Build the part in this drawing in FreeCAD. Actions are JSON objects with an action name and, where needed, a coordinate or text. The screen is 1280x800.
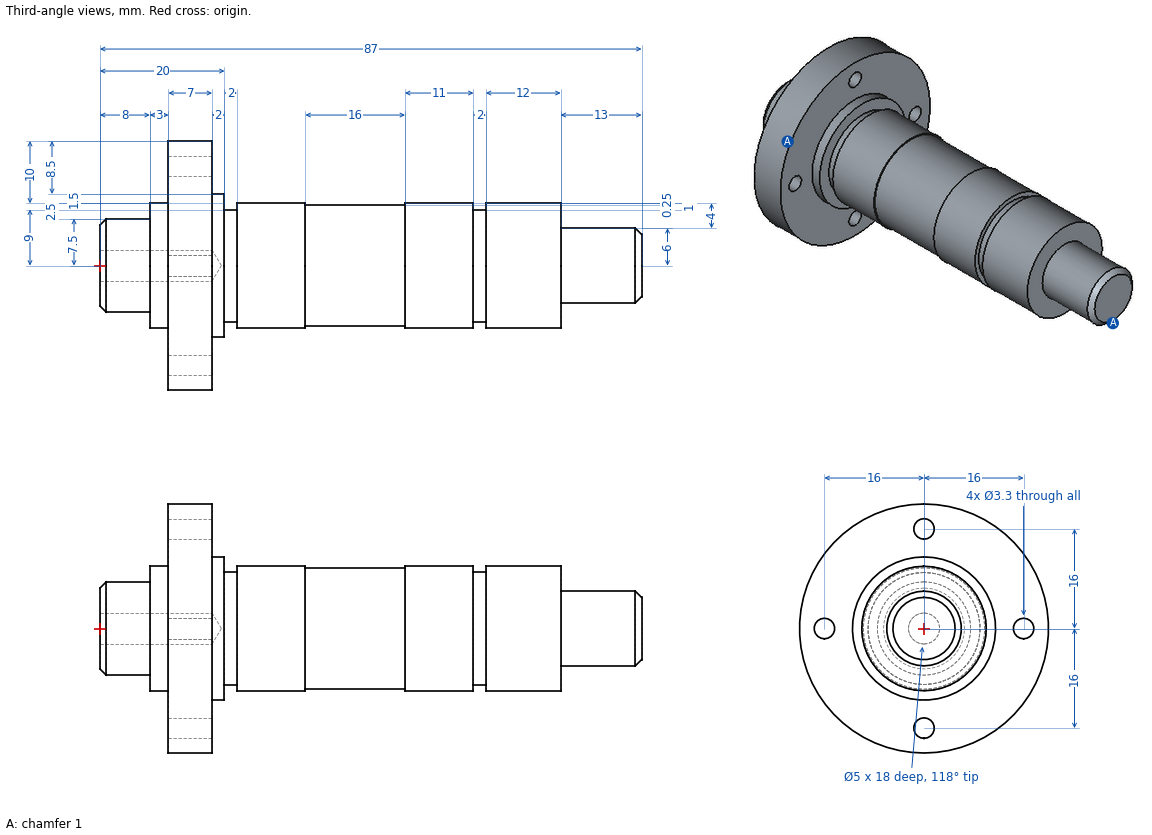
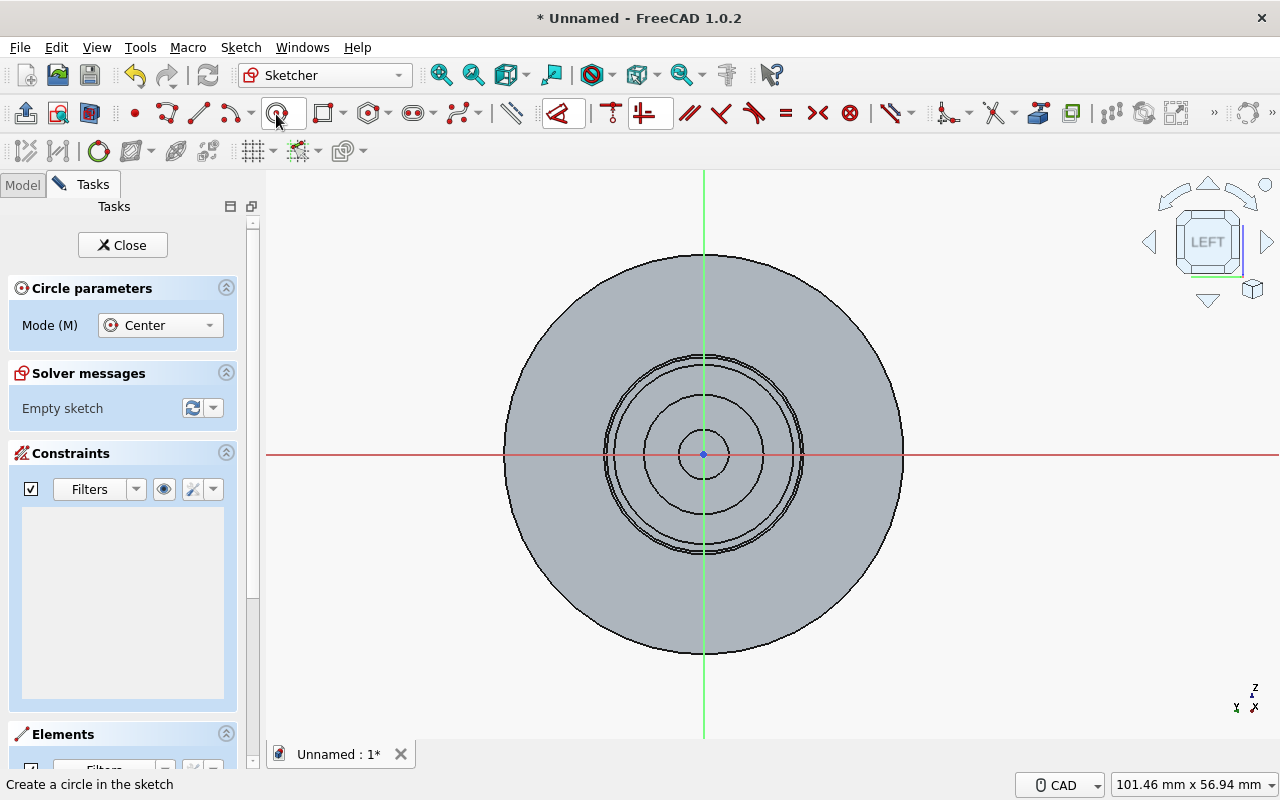
{"action": "scroll", "coordinate": [544, 454], "scroll_direction": "up", "scroll_amount": 2}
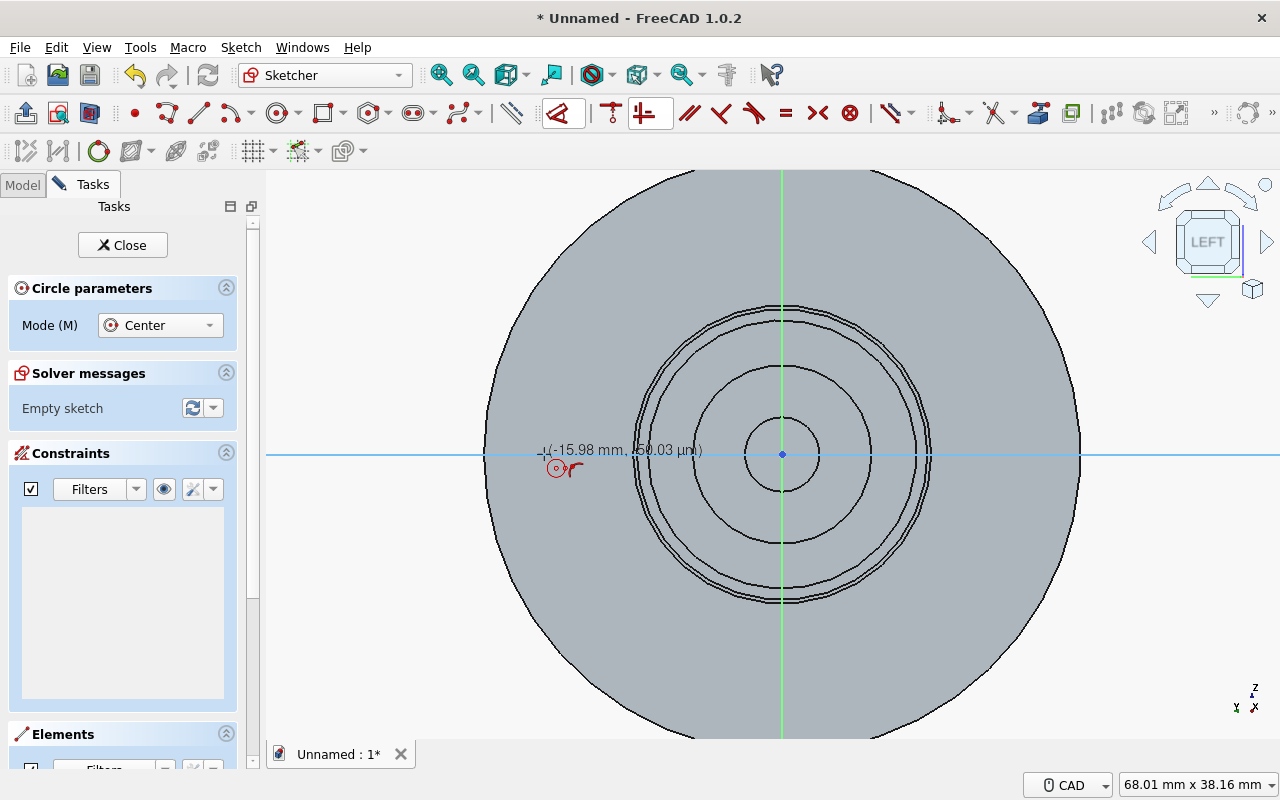
{"action": "left_click", "coordinate": [544, 454]}
{"action": "mouse_move", "coordinate": [561, 437]}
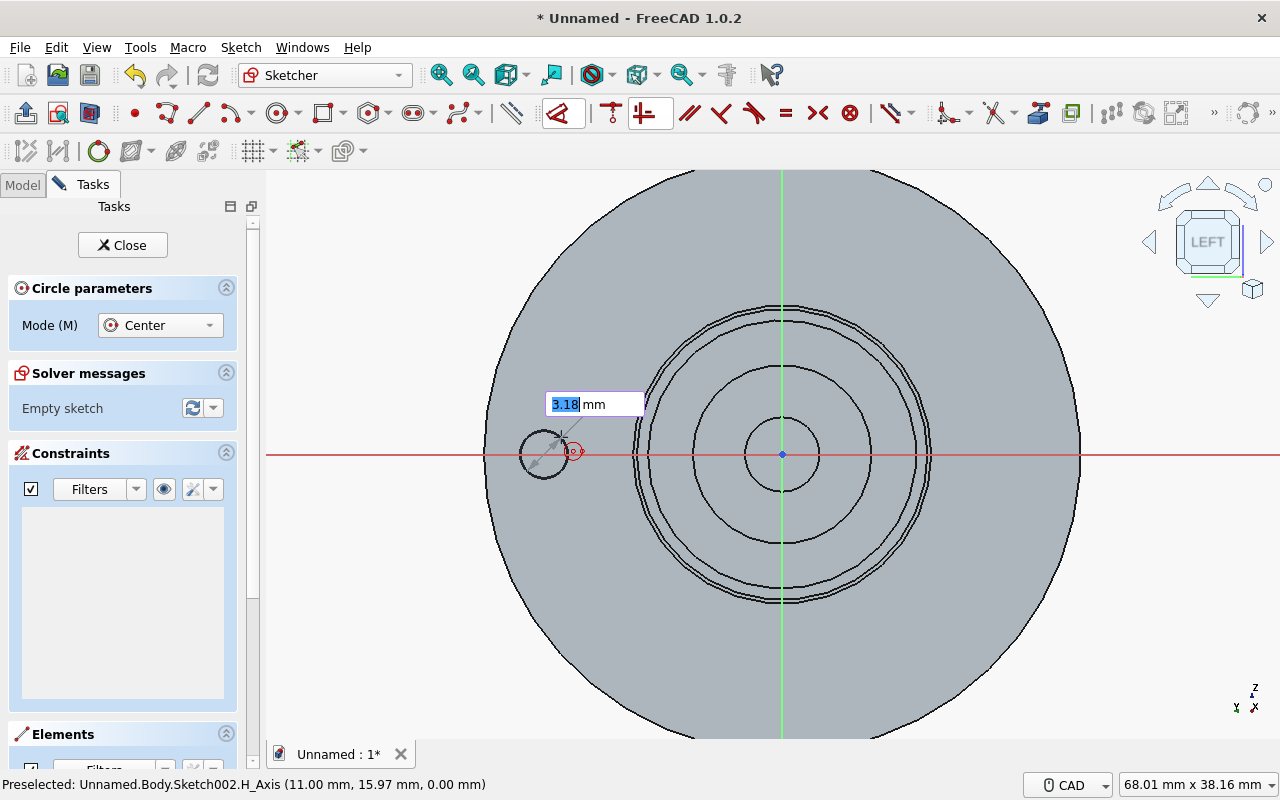
{"action": "type", "text": "3.3"}
{"action": "key", "text": "Return"}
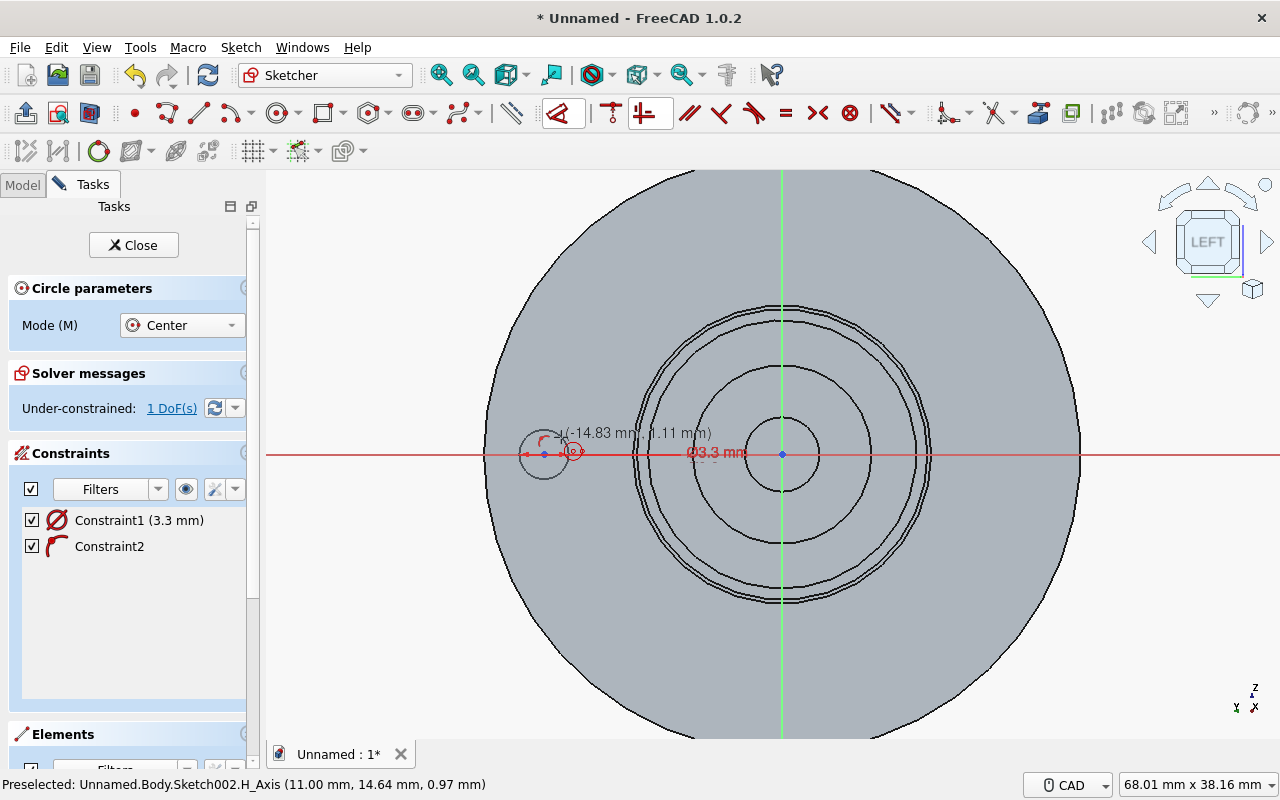
{"action": "left_click", "coordinate": [782, 693]}
{"action": "mouse_move", "coordinate": [800, 676]}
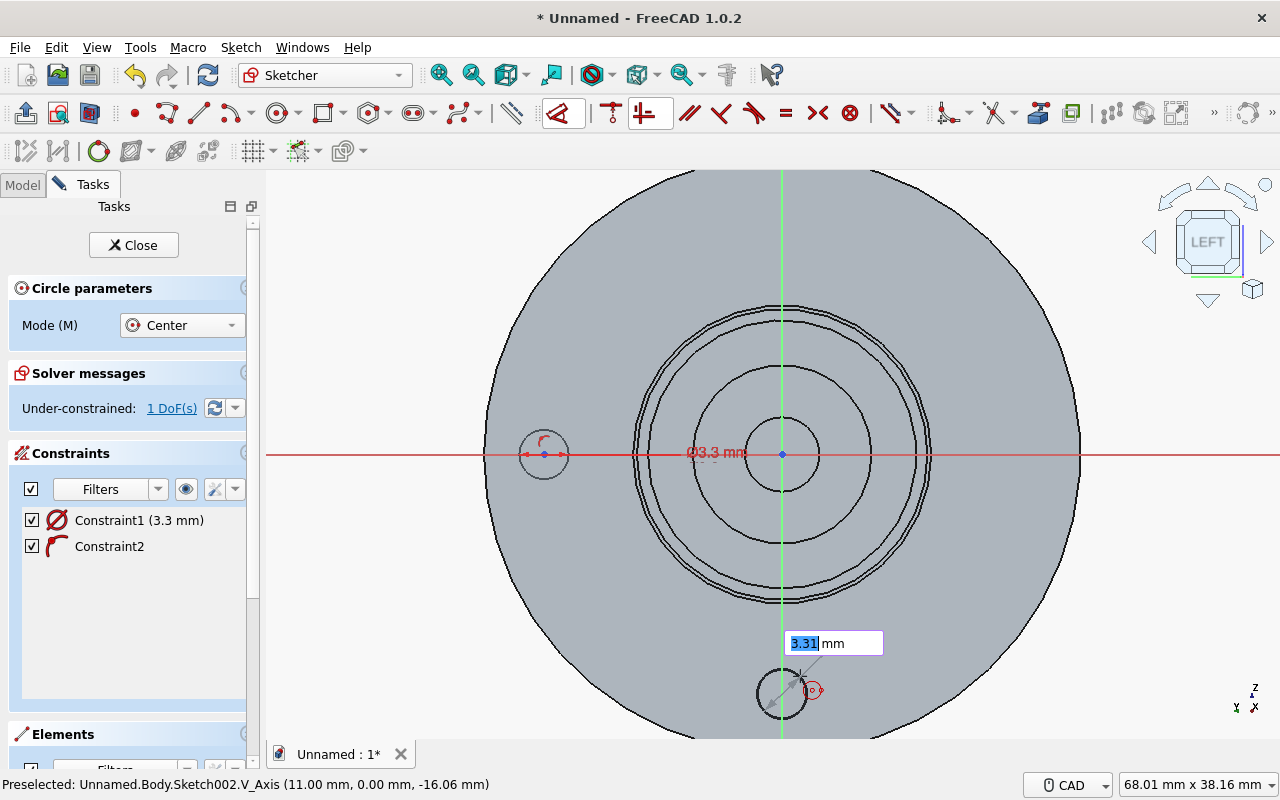
{"action": "type", "text": "3.3"}
{"action": "key", "text": "Return"}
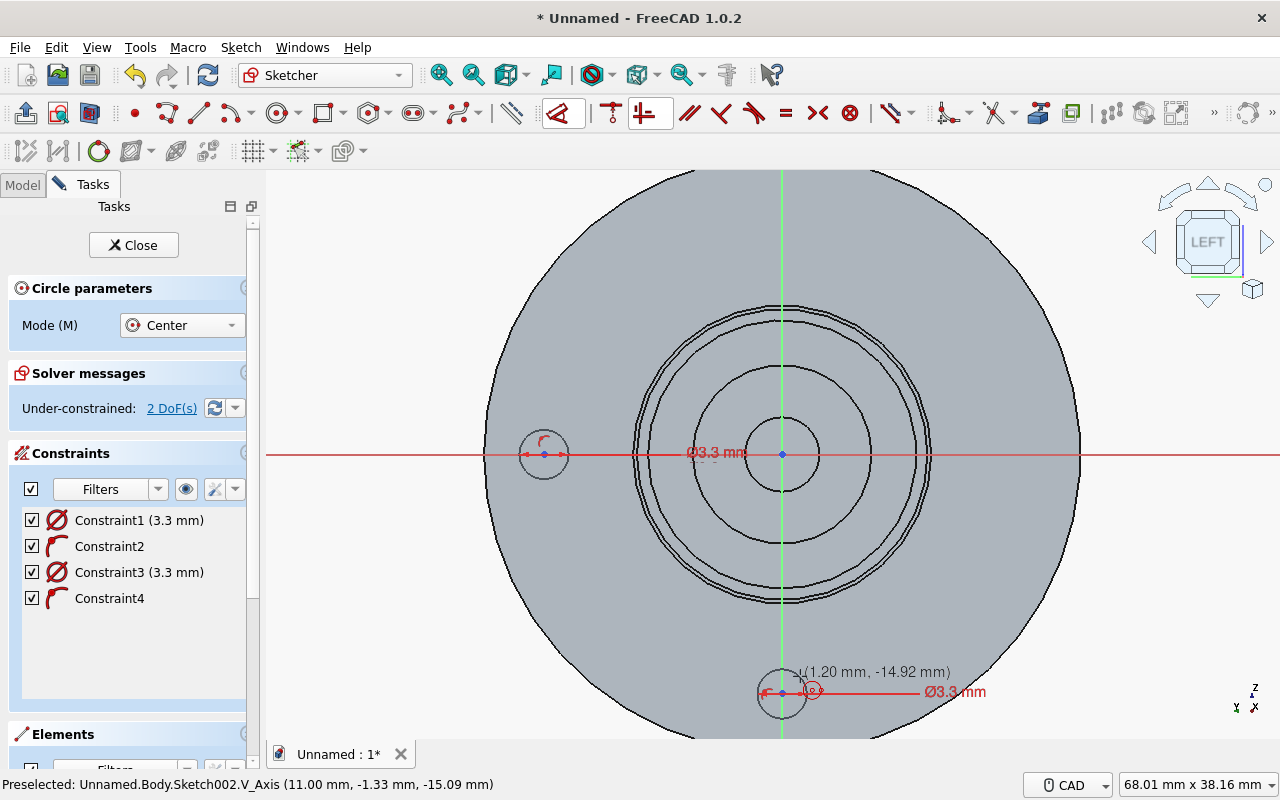
{"action": "left_click", "coordinate": [1021, 454]}
{"action": "mouse_move", "coordinate": [1038, 437]}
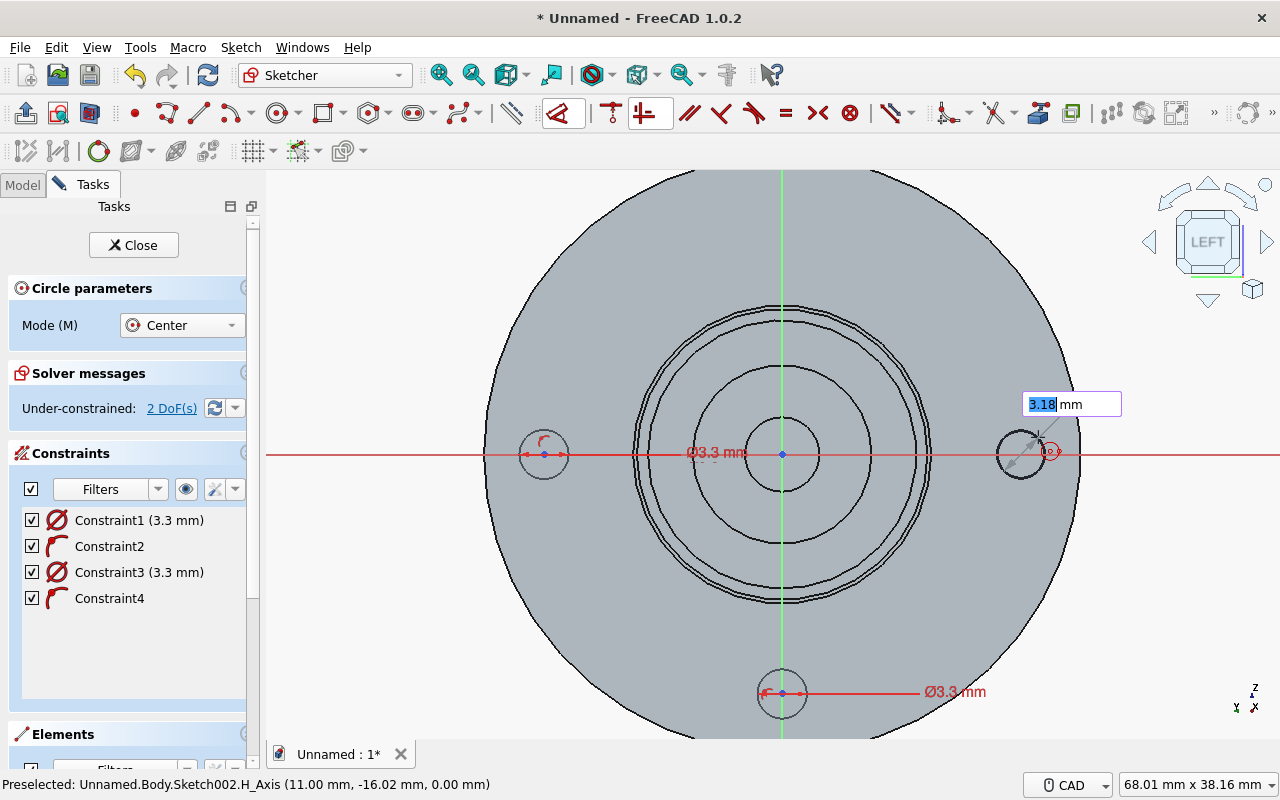
{"action": "type", "text": "3.3"}
{"action": "key", "text": "Return"}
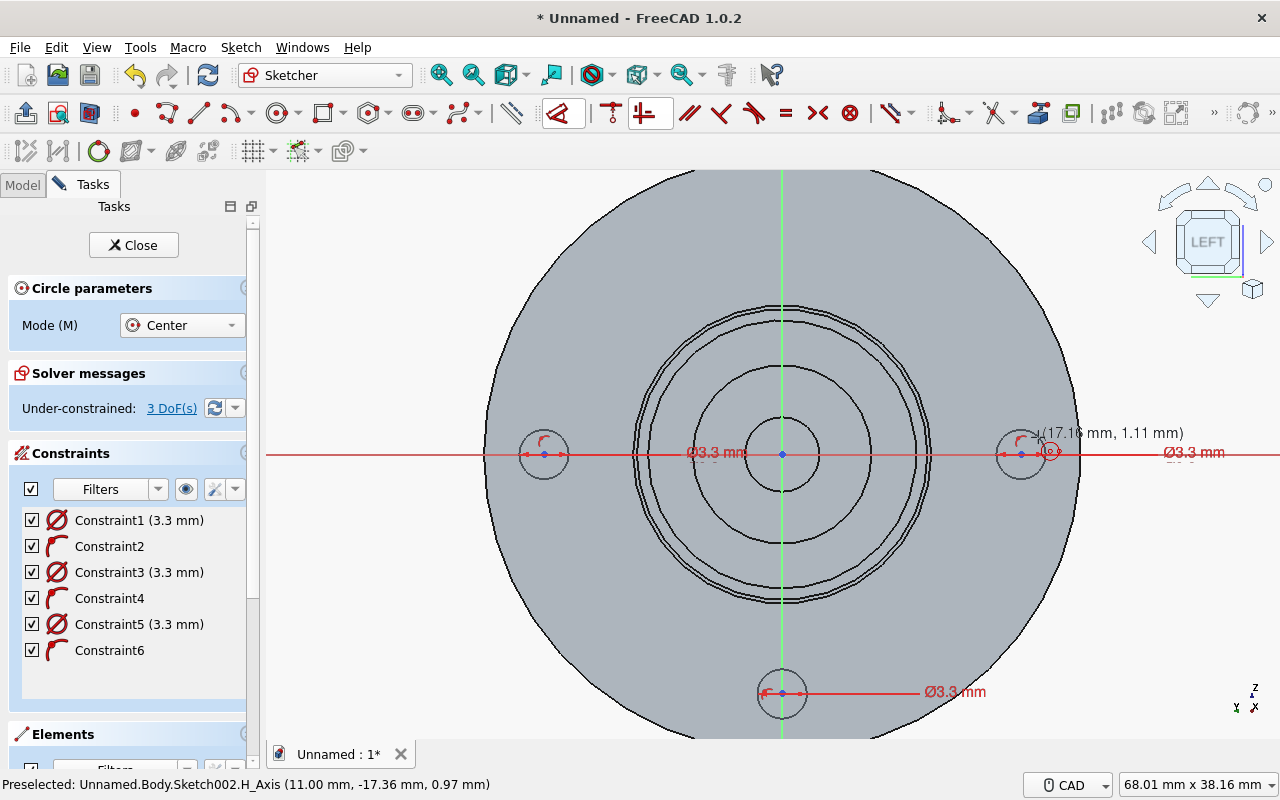
{"action": "left_click", "coordinate": [782, 216]}
{"action": "mouse_move", "coordinate": [800, 199]}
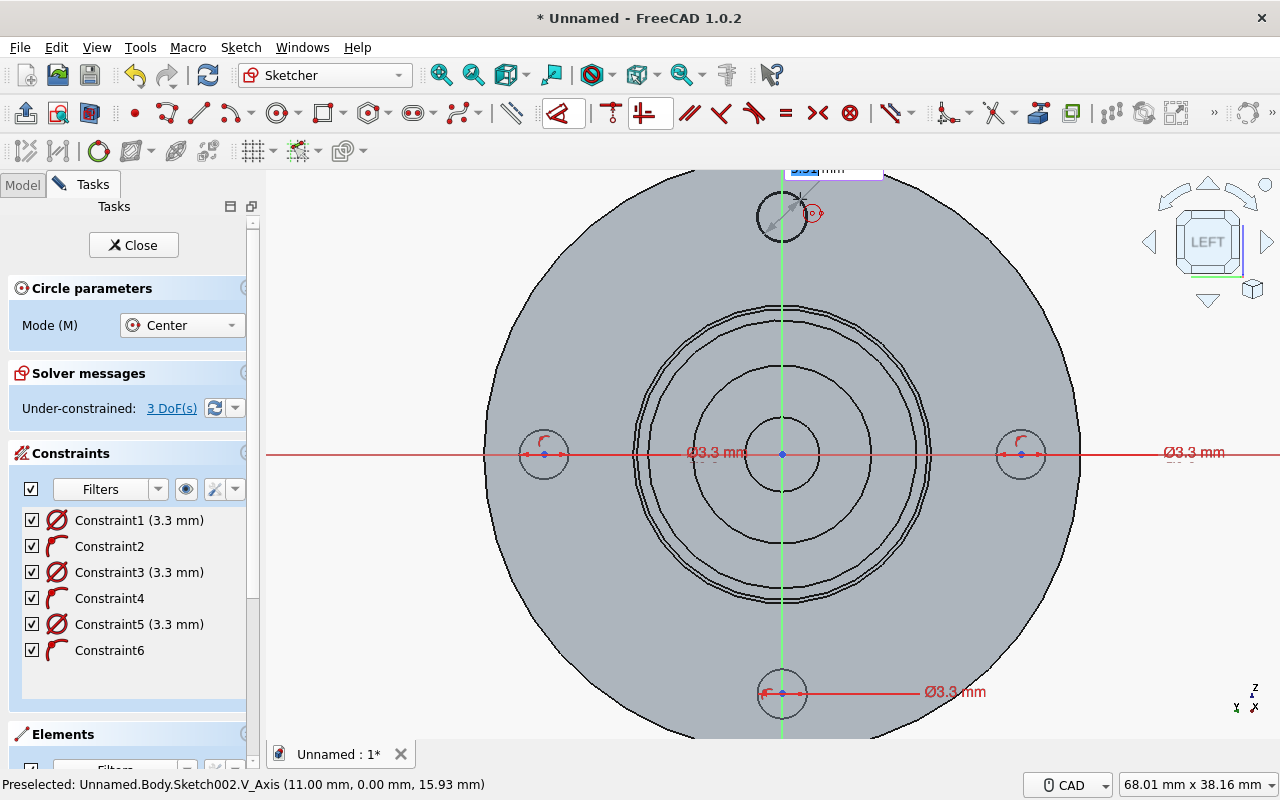
{"action": "type", "text": "3.3"}
{"action": "key", "text": "Return"}
{"action": "key", "text": "Escape"}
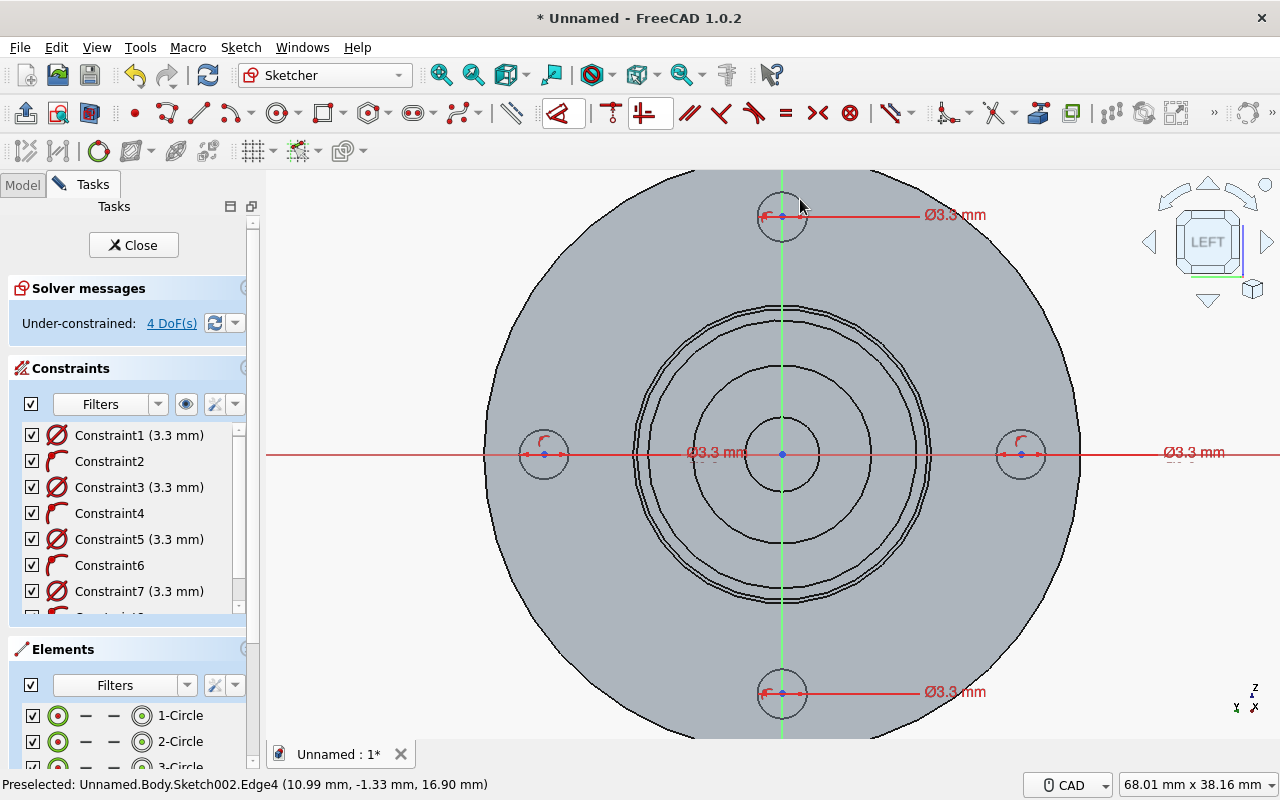
{"action": "left_click", "coordinate": [544, 454]}